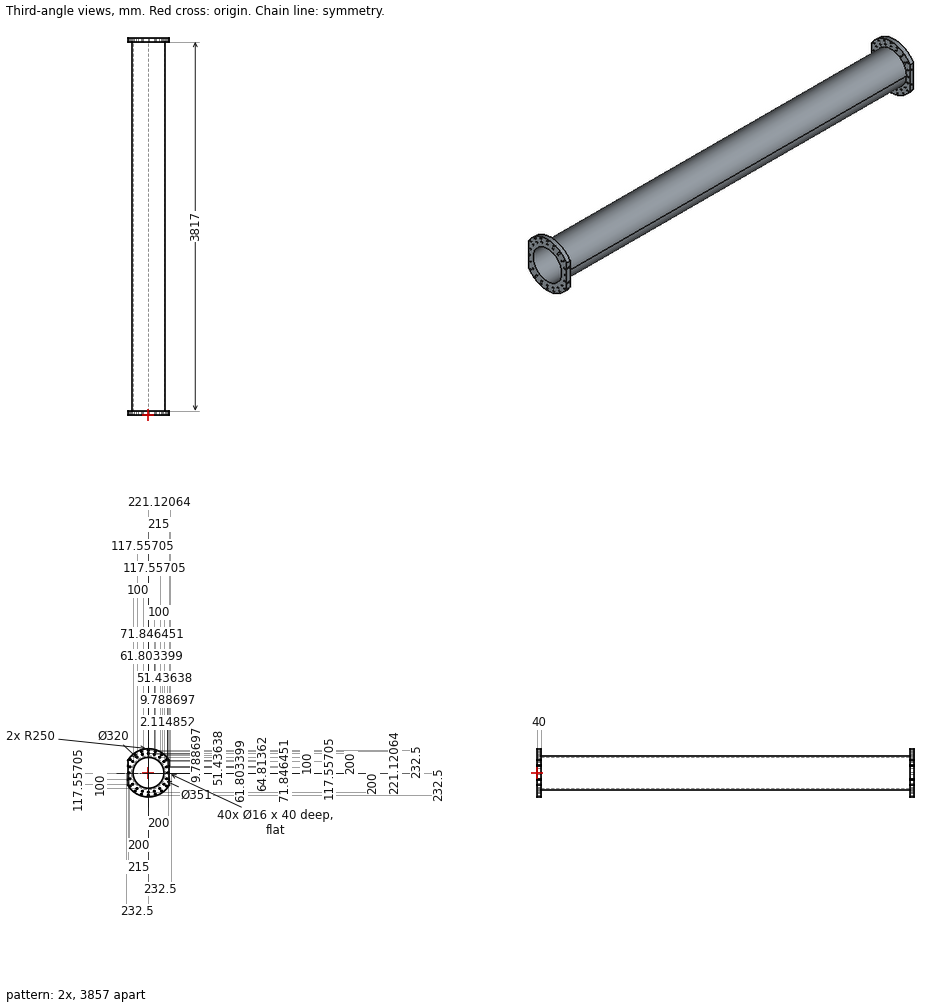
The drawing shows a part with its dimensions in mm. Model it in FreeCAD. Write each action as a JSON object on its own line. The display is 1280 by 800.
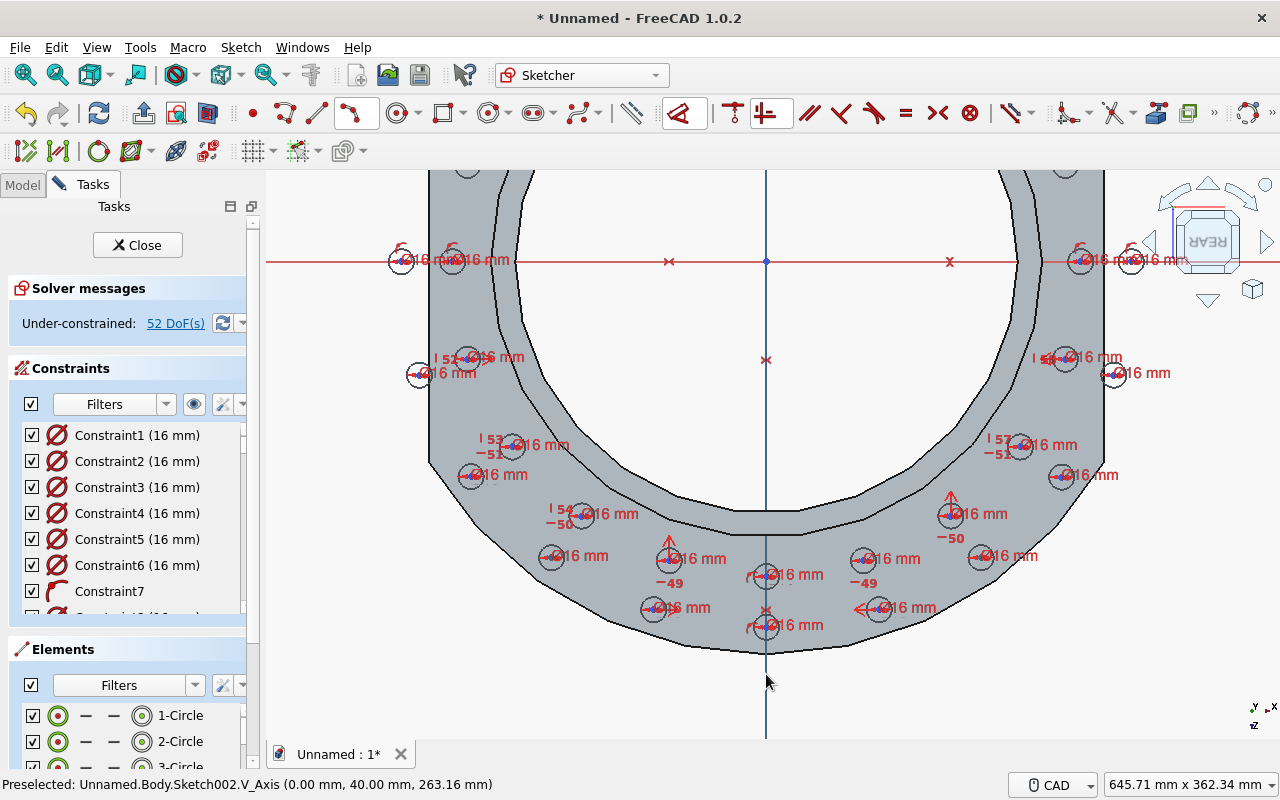
{"action": "key", "text": "s"}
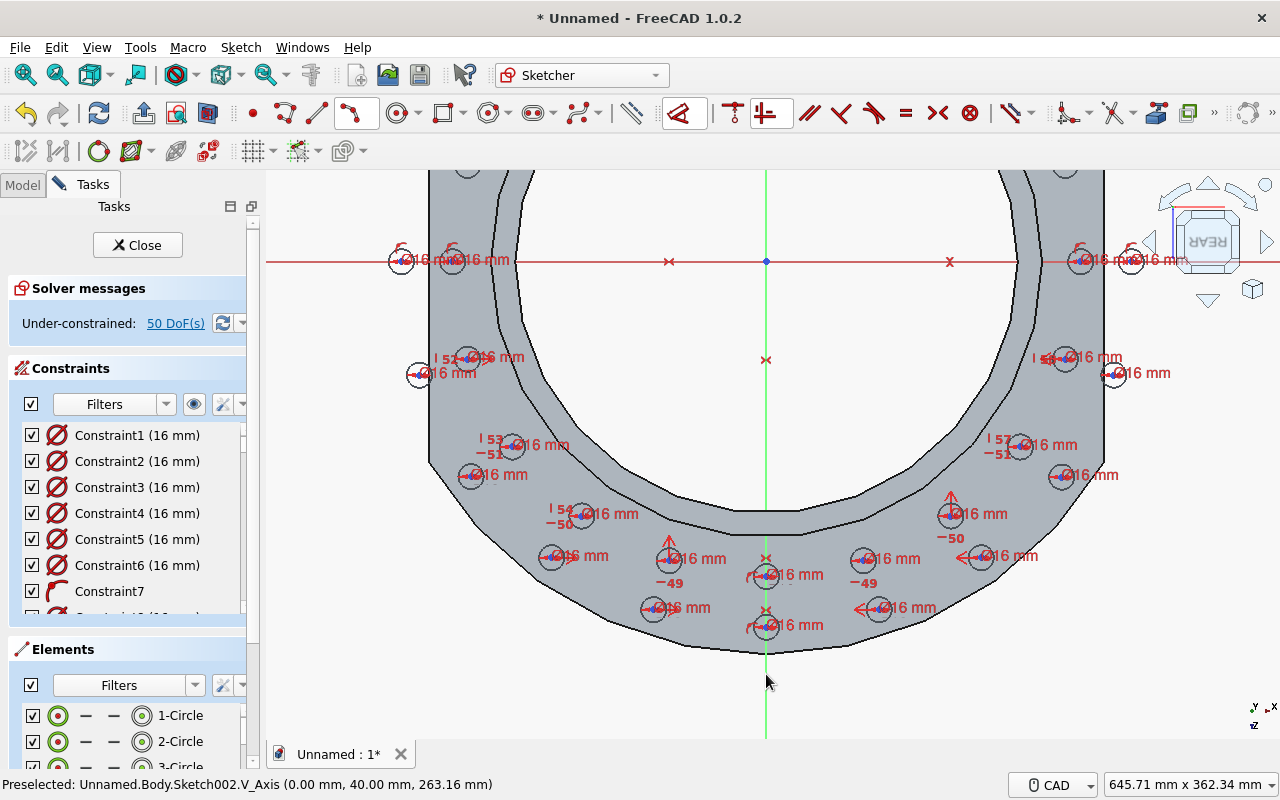
{"action": "left_click", "coordinate": [1062, 477]}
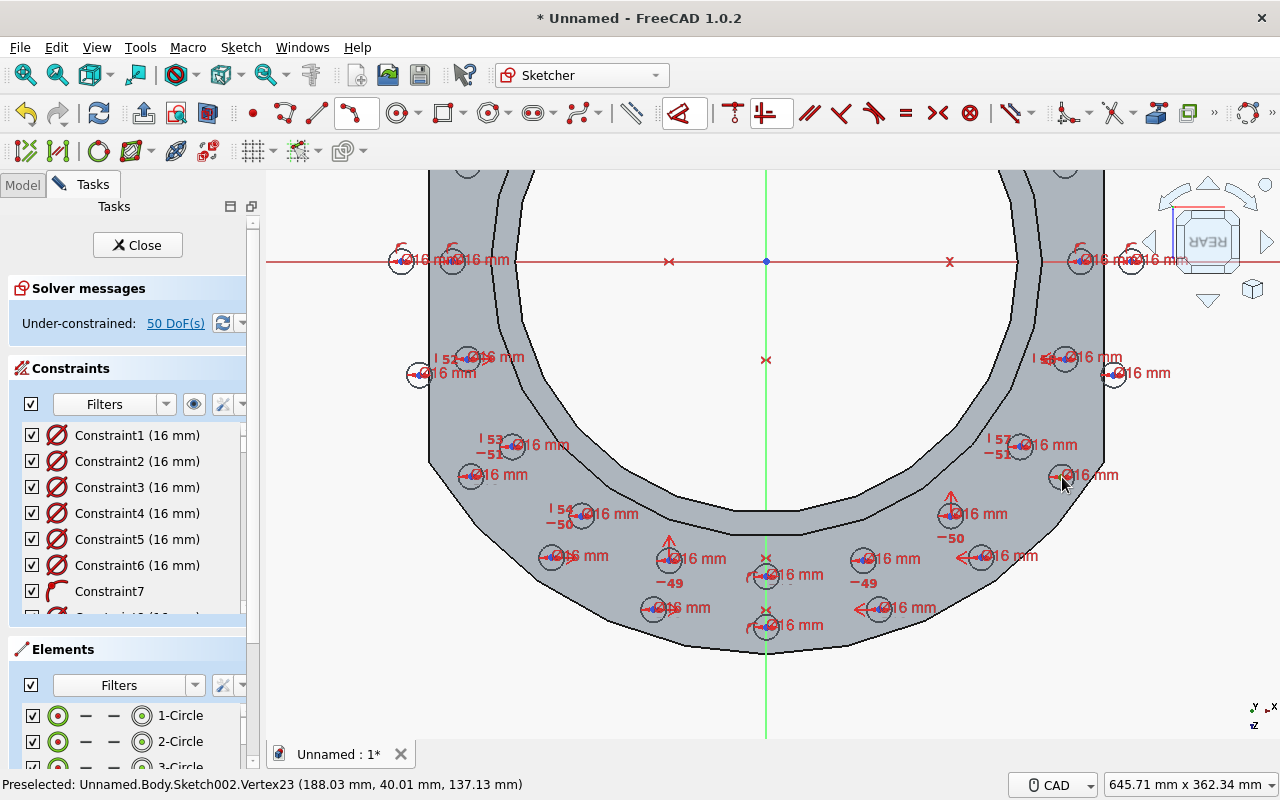
{"action": "left_click", "coordinate": [471, 477]}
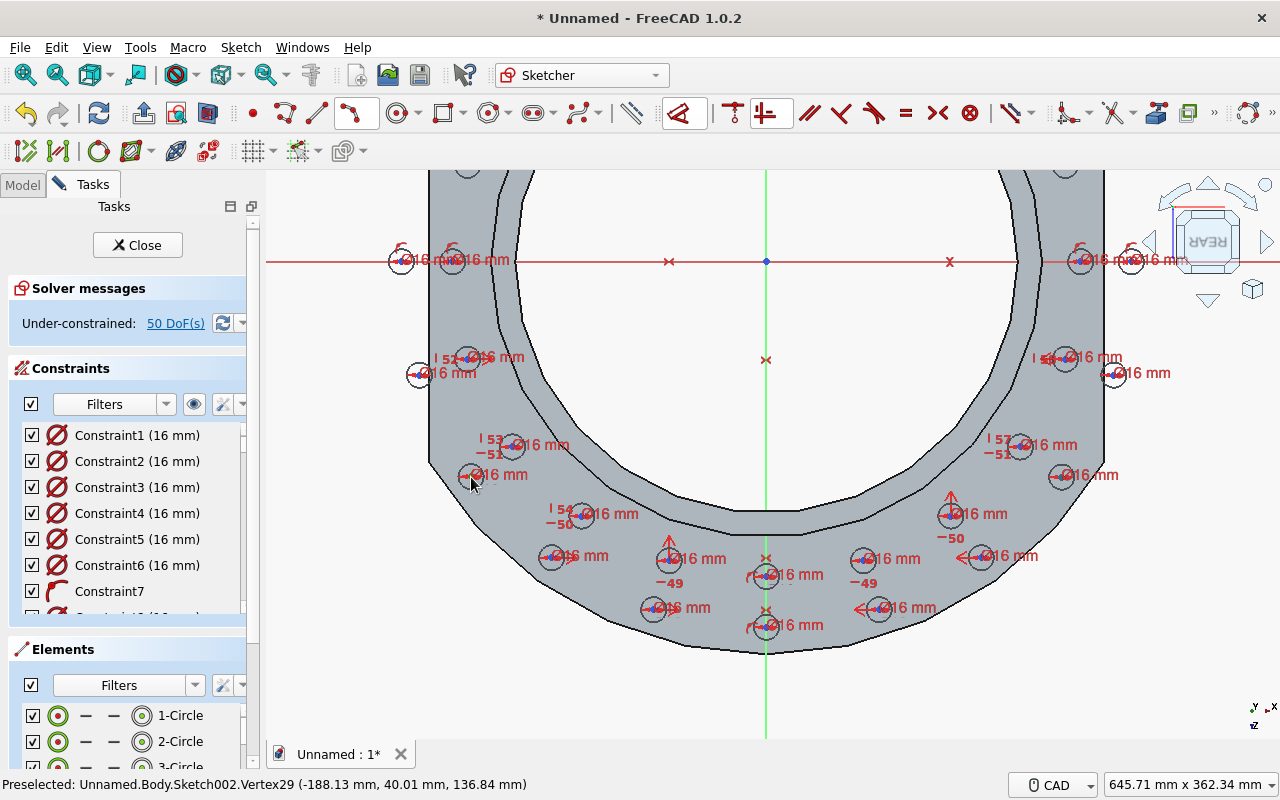
{"action": "left_click", "coordinate": [766, 674]}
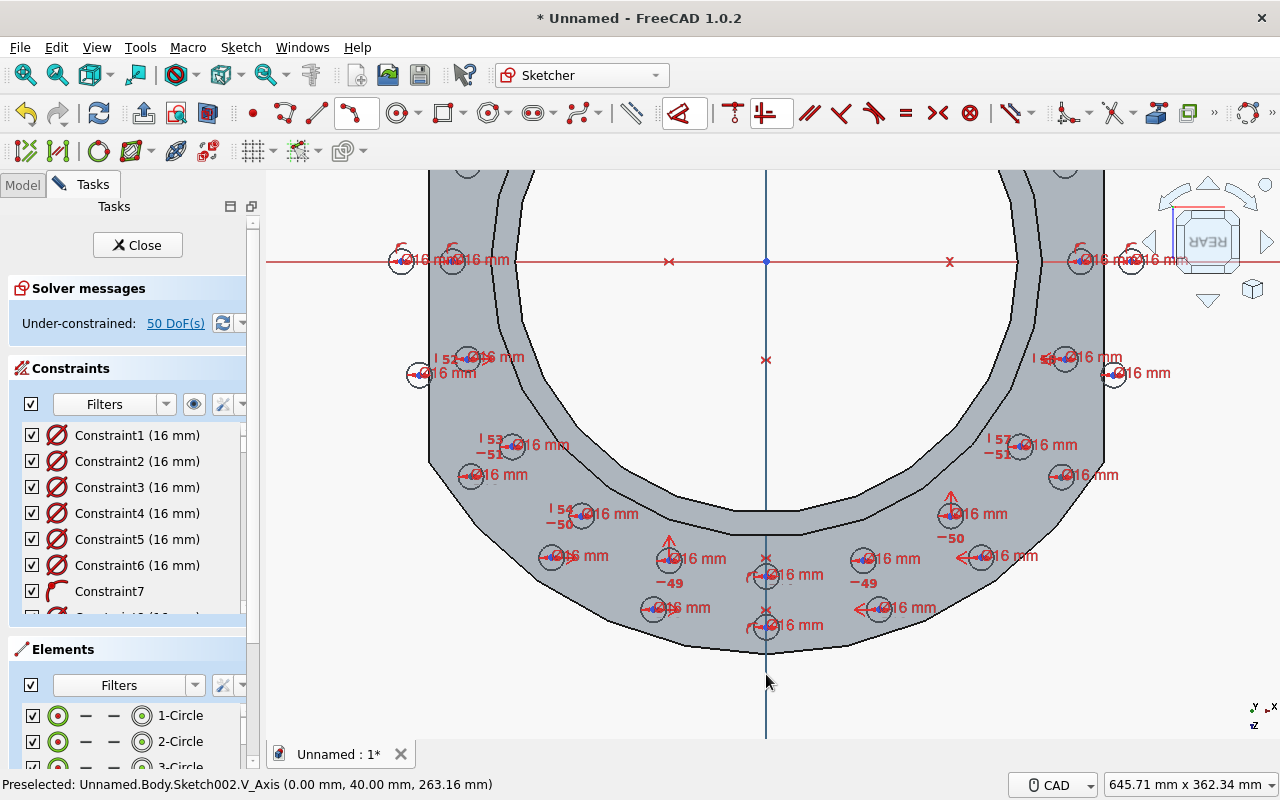
{"action": "left_click", "coordinate": [938, 114]}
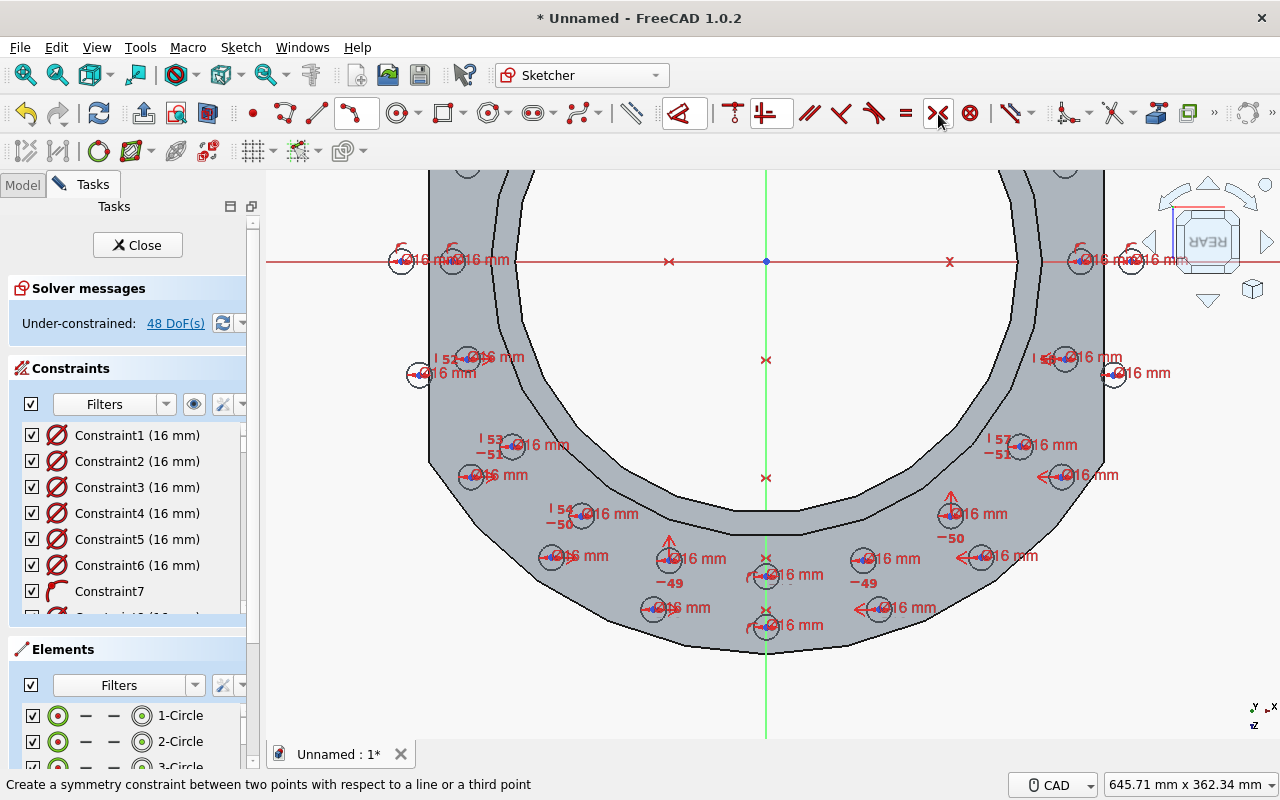
{"action": "left_click", "coordinate": [1114, 375]}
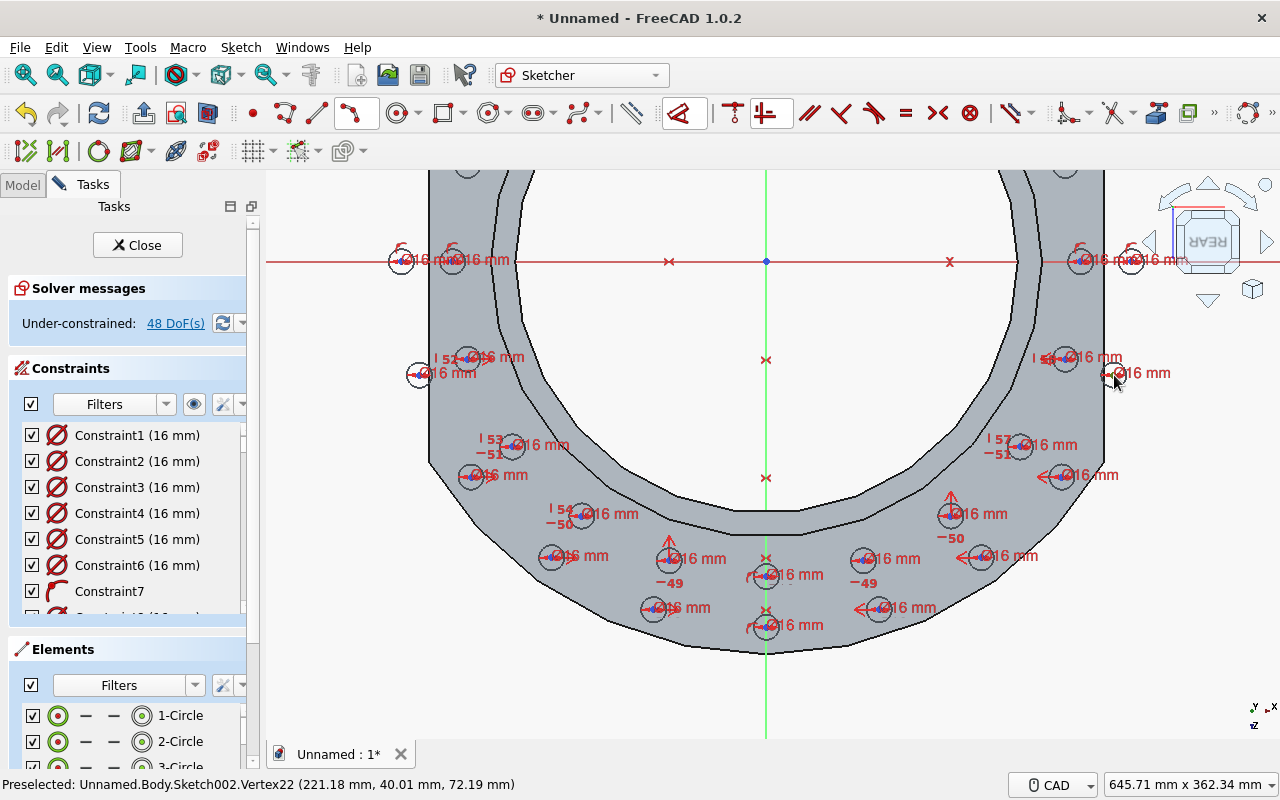
{"action": "left_click", "coordinate": [419, 375]}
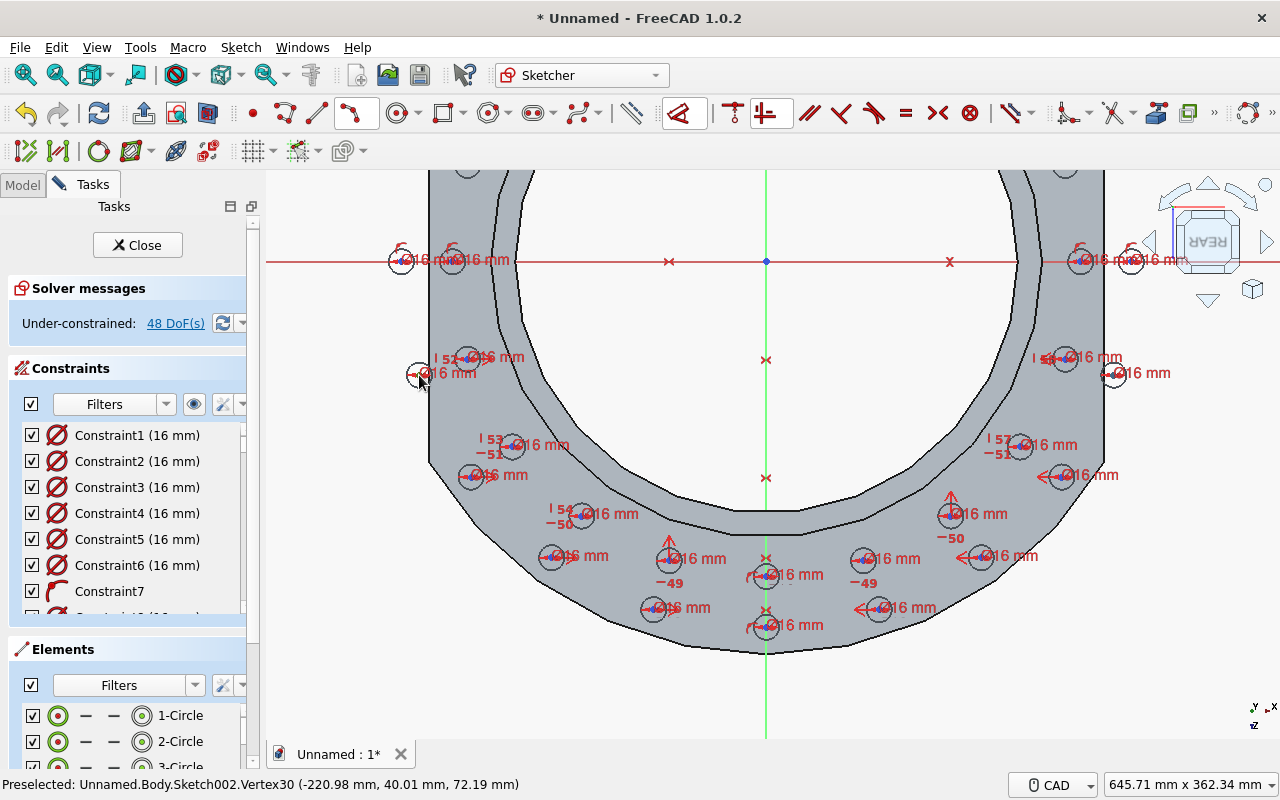
{"action": "left_click", "coordinate": [766, 674]}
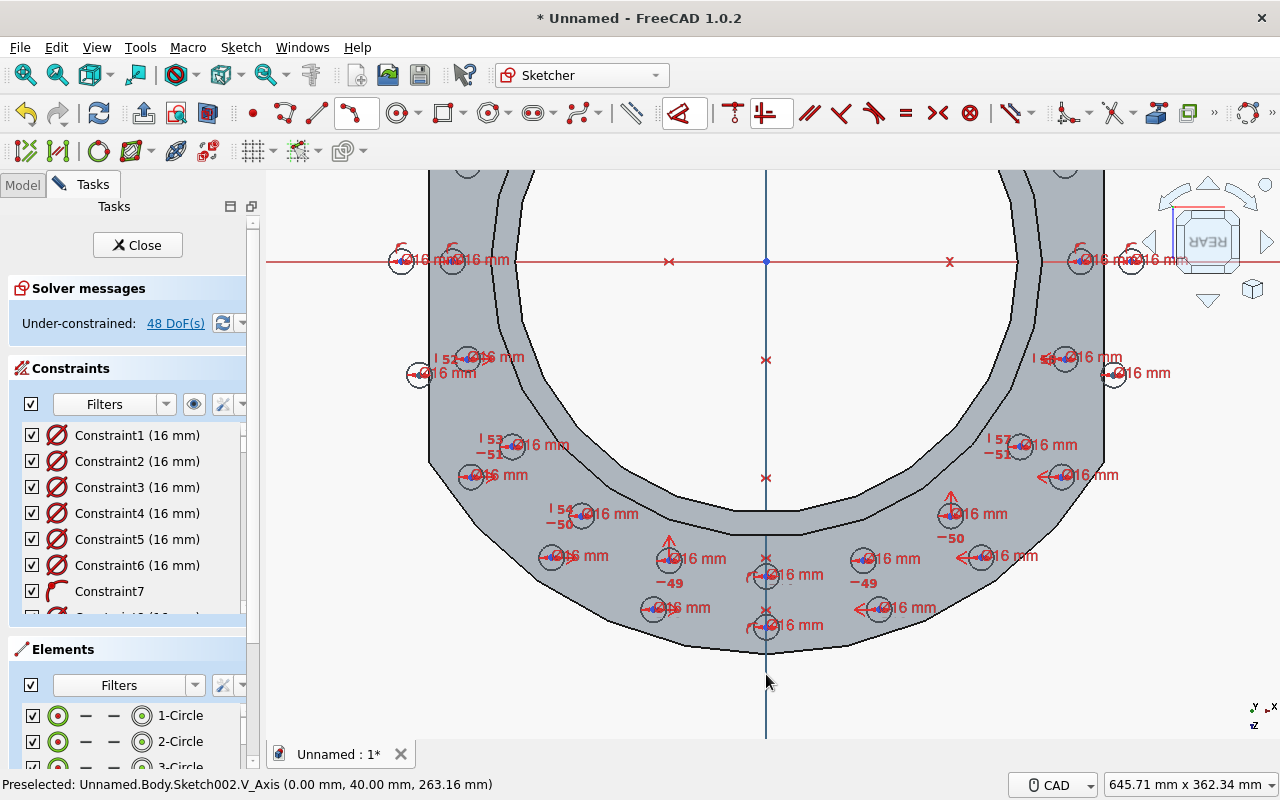
{"action": "left_click", "coordinate": [938, 114]}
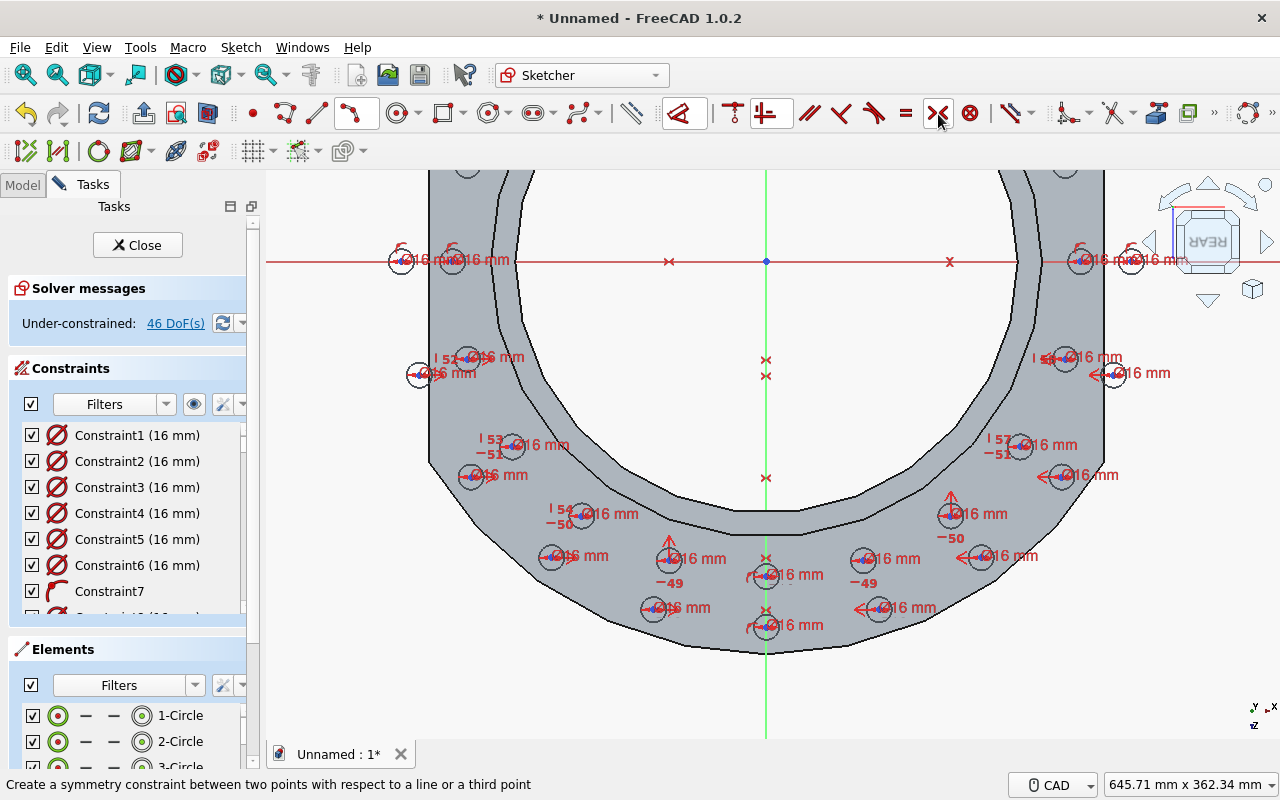
{"action": "left_click", "coordinate": [419, 375]}